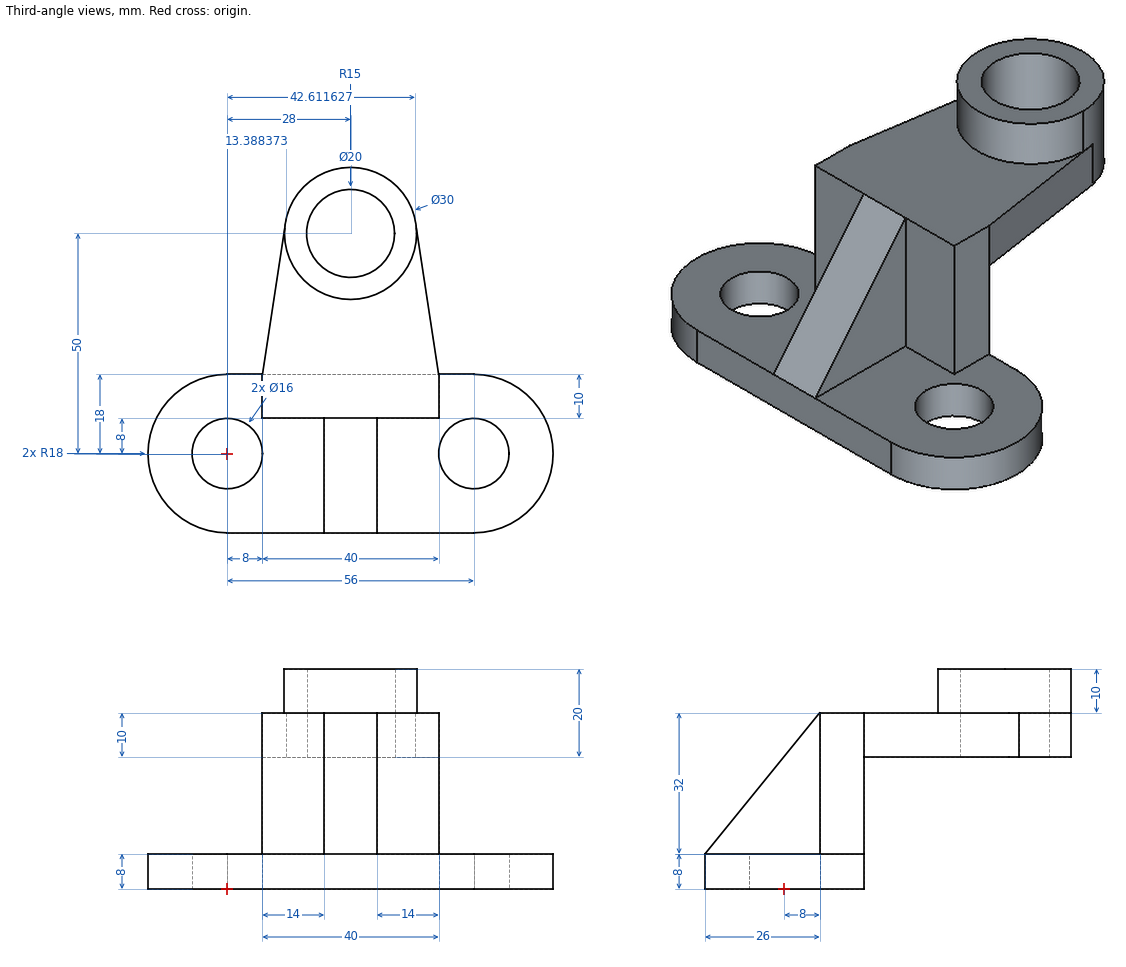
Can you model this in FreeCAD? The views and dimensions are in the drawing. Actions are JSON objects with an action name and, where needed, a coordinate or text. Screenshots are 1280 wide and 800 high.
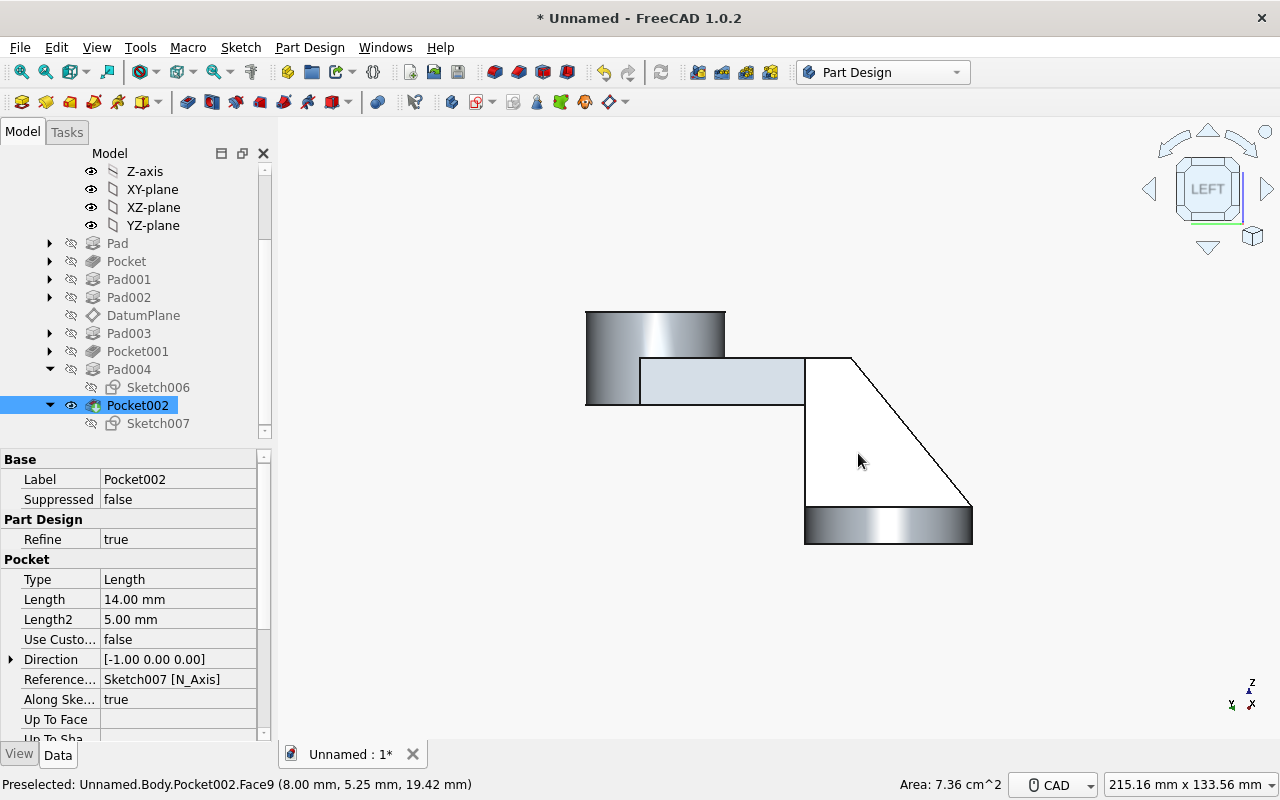
{"action": "left_click", "coordinate": [476, 102]}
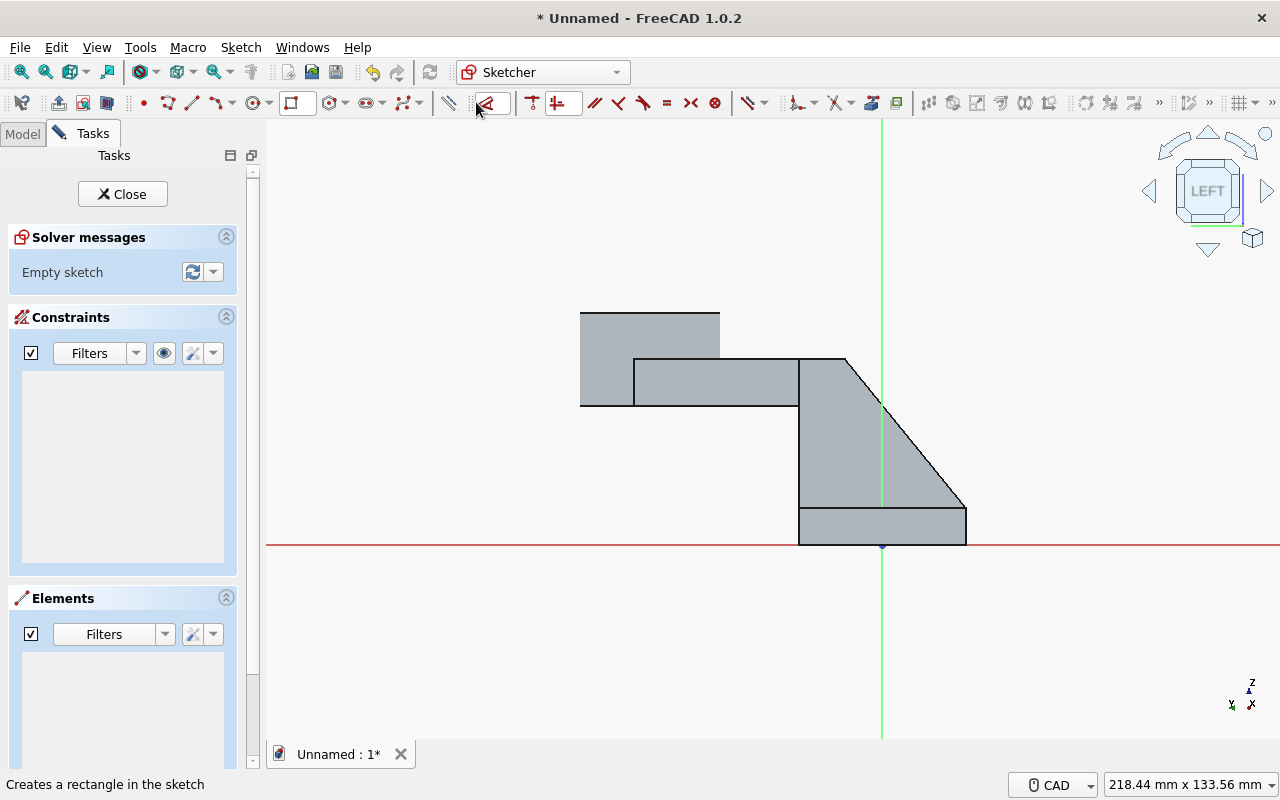
{"action": "scroll", "coordinate": [1069, 471], "scroll_direction": "up", "scroll_amount": 4}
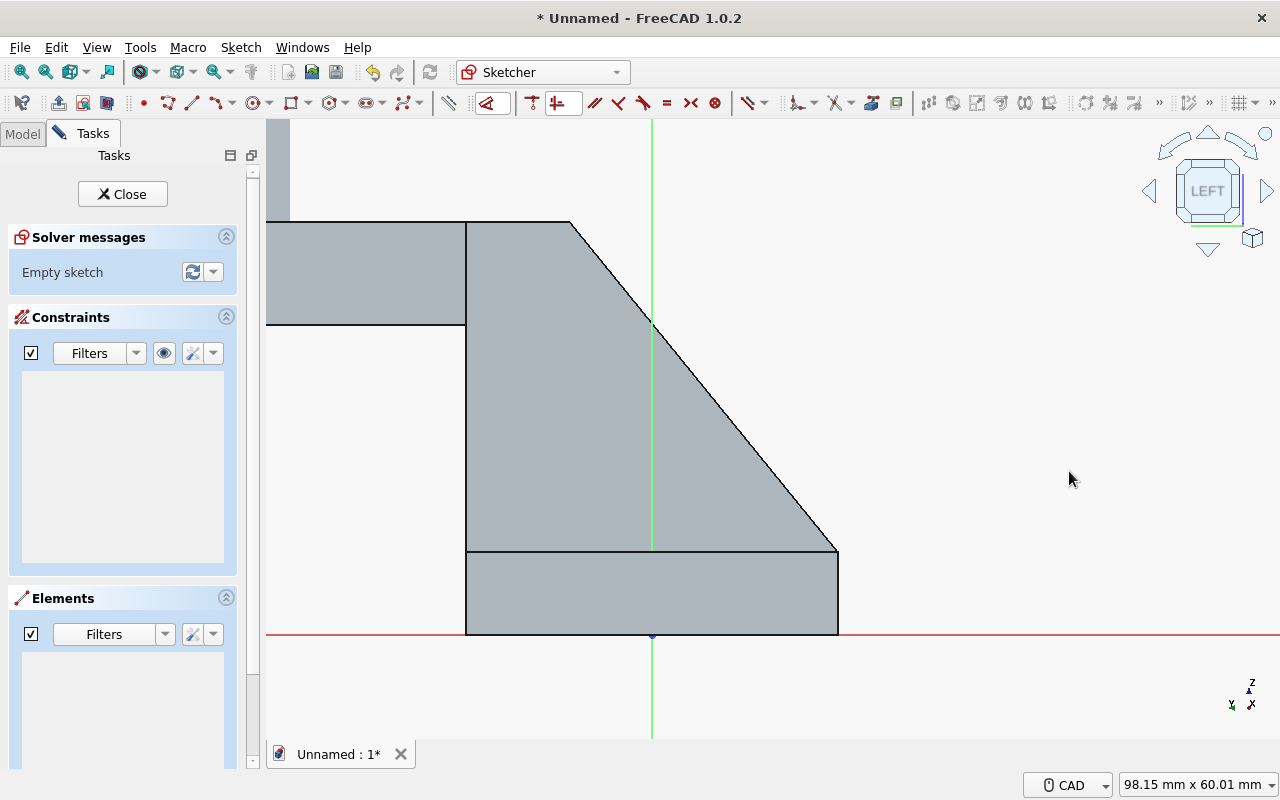
{"action": "left_click", "coordinate": [168, 104]}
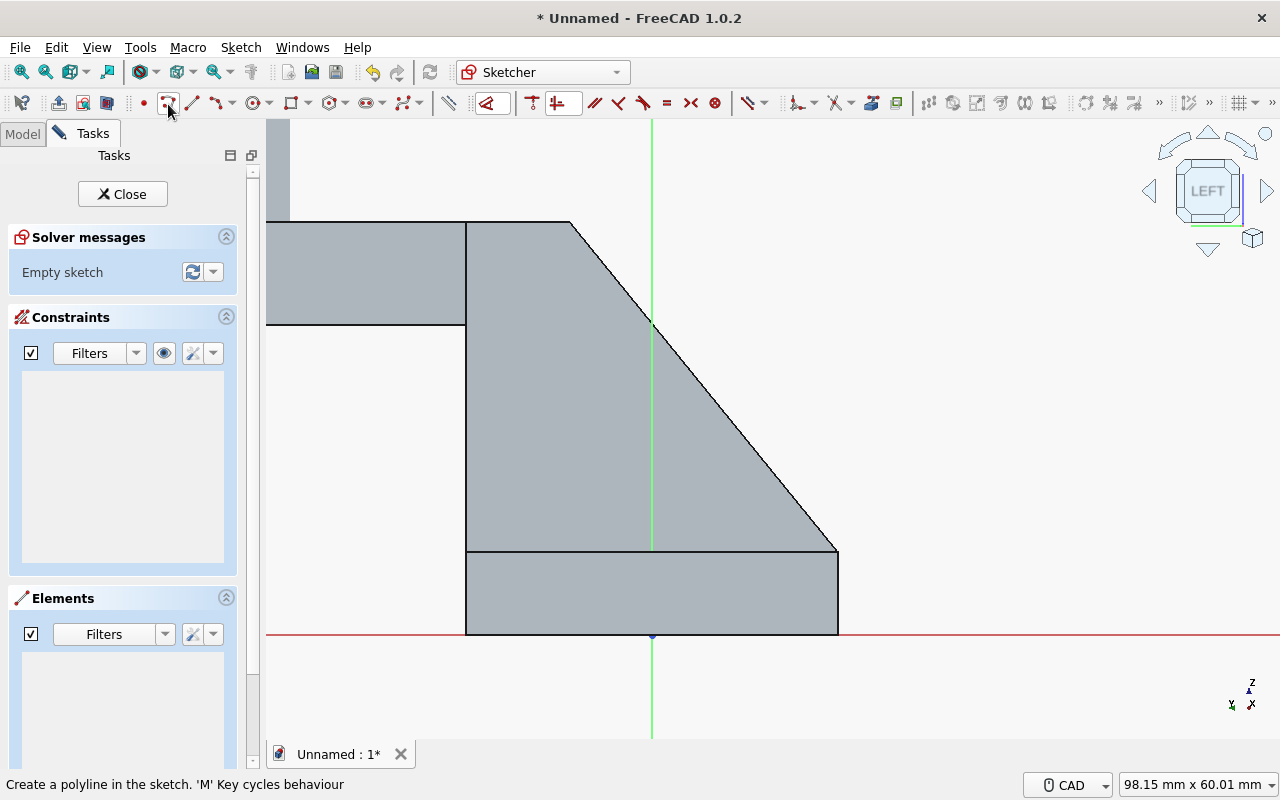
{"action": "left_click", "coordinate": [569, 552]}
{"action": "left_click", "coordinate": [838, 552]}
{"action": "left_click", "coordinate": [569, 222]}
{"action": "left_click", "coordinate": [569, 553]}
{"action": "key", "text": "Escape"}
{"action": "key", "text": "Escape"}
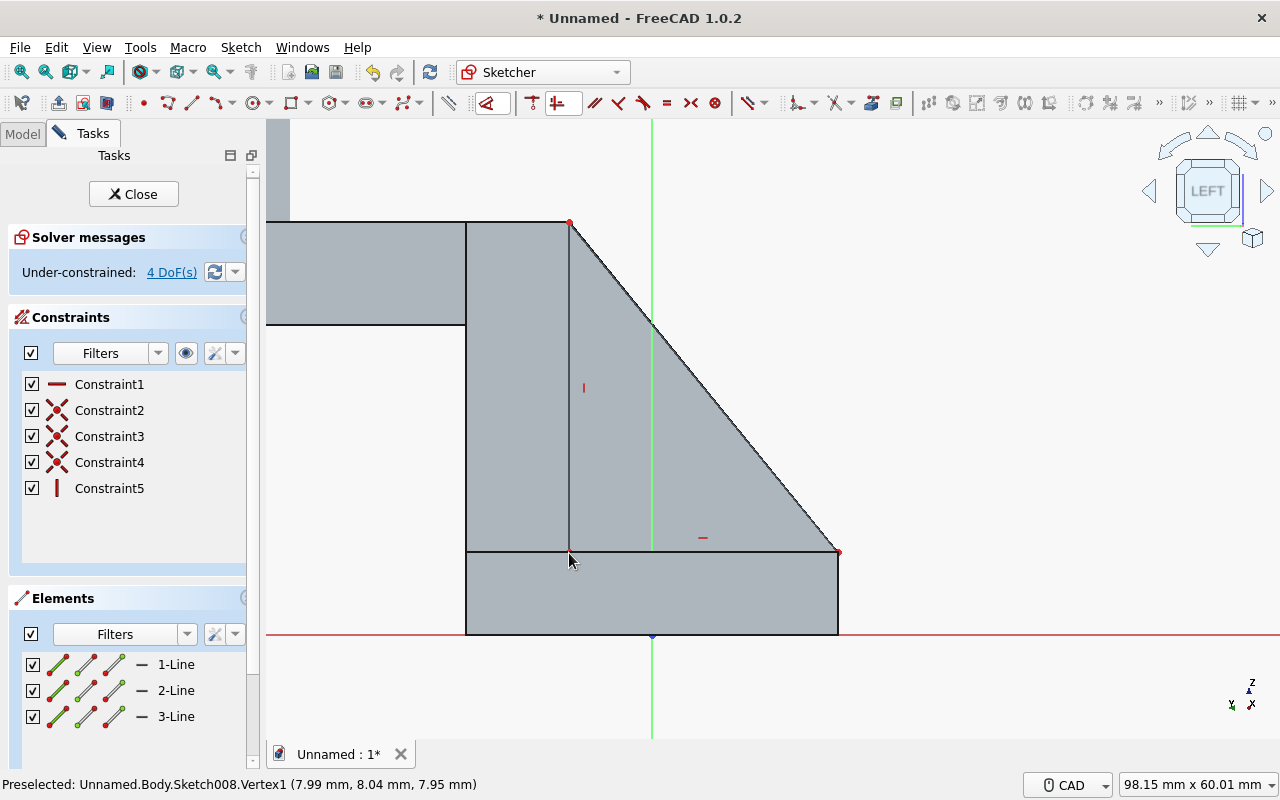
{"action": "left_click", "coordinate": [650, 553]}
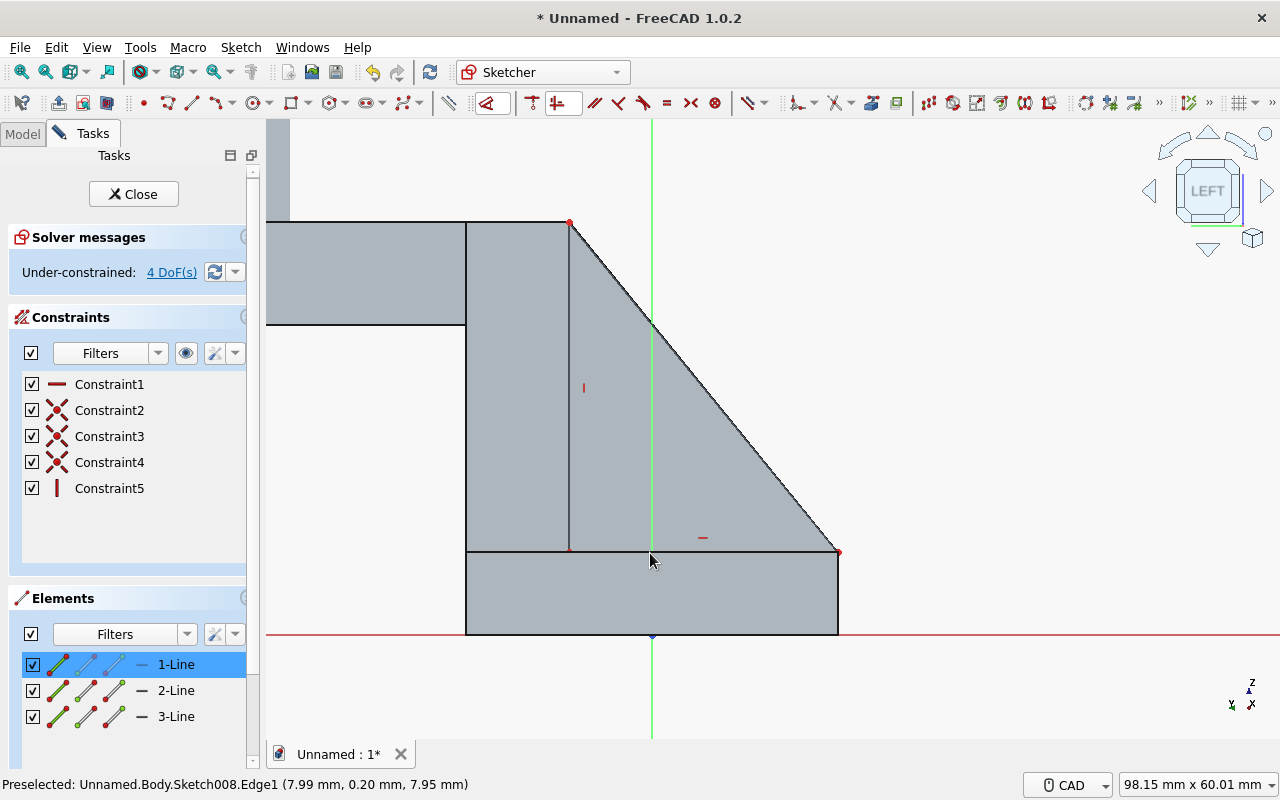
{"action": "left_click", "coordinate": [504, 104]}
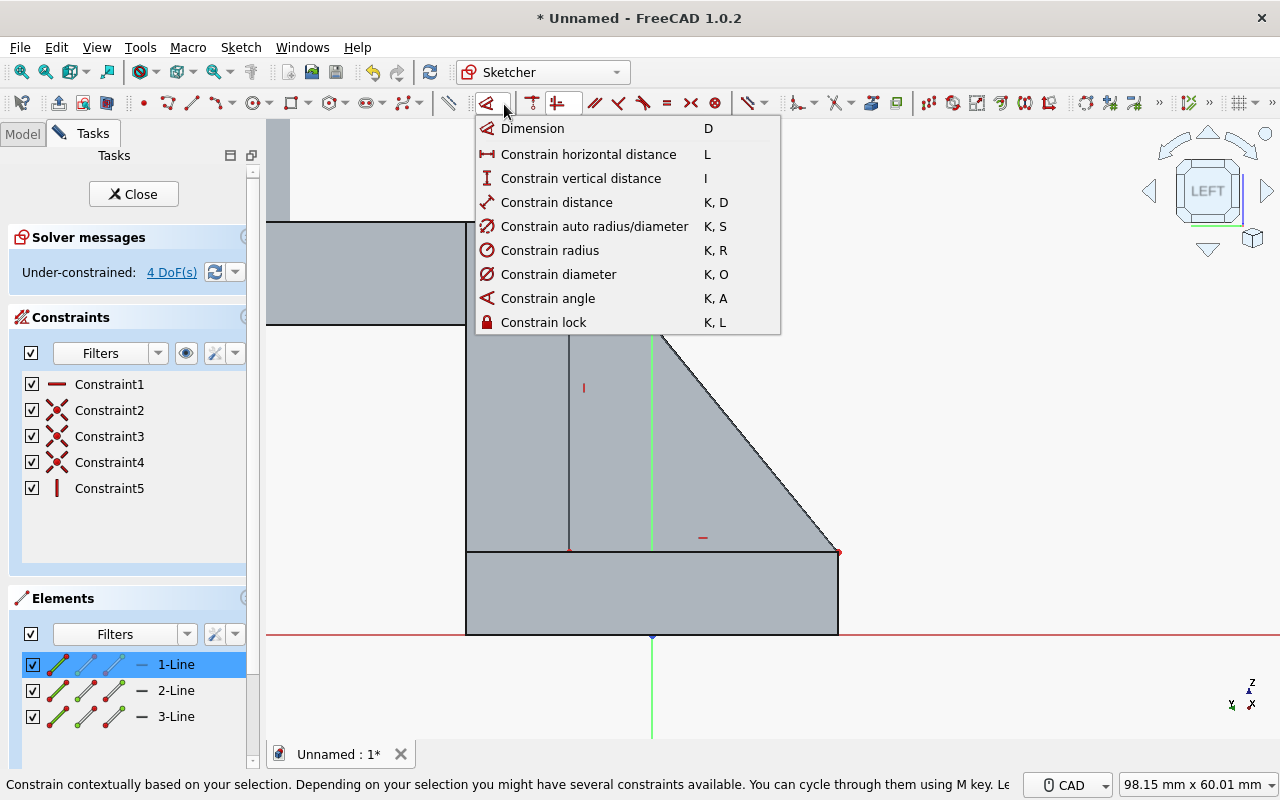
{"action": "left_click", "coordinate": [628, 154]}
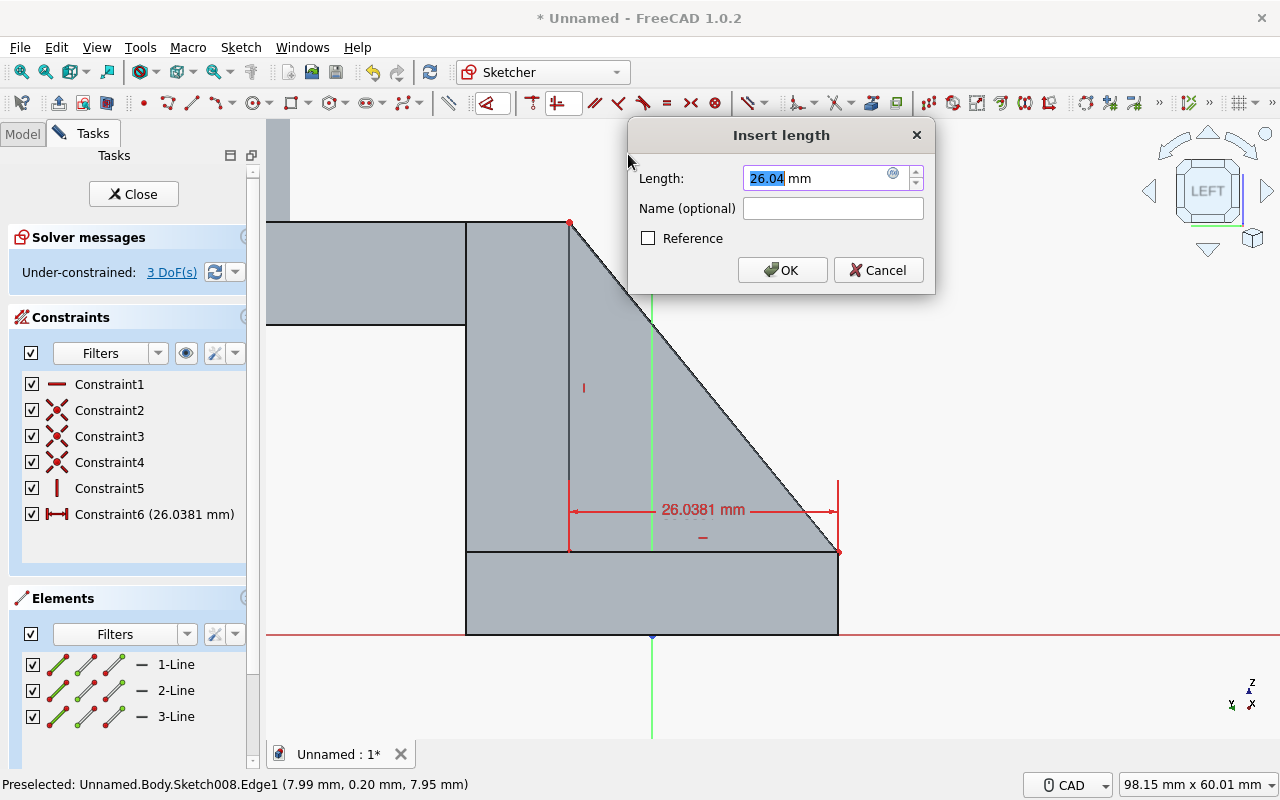
{"action": "type", "text": "26"}
{"action": "key", "text": "Return"}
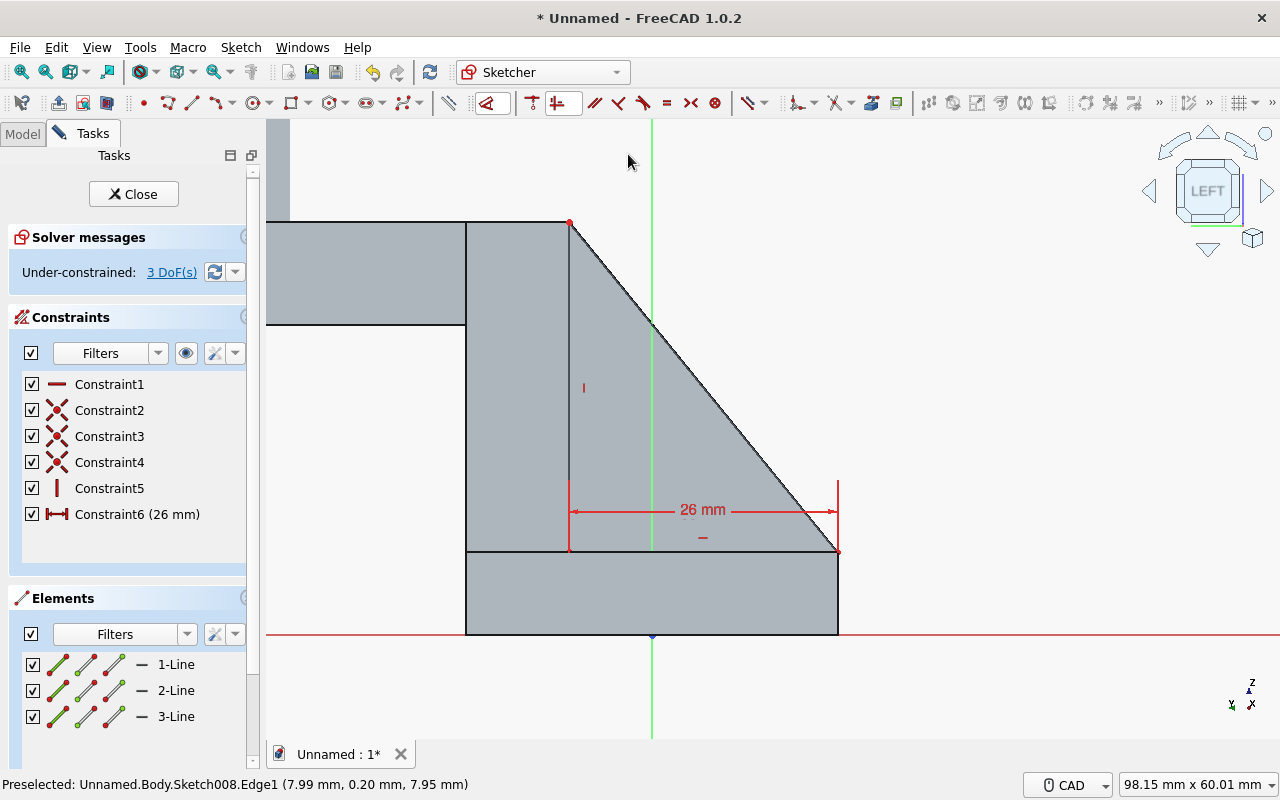
{"action": "left_click", "coordinate": [569, 322]}